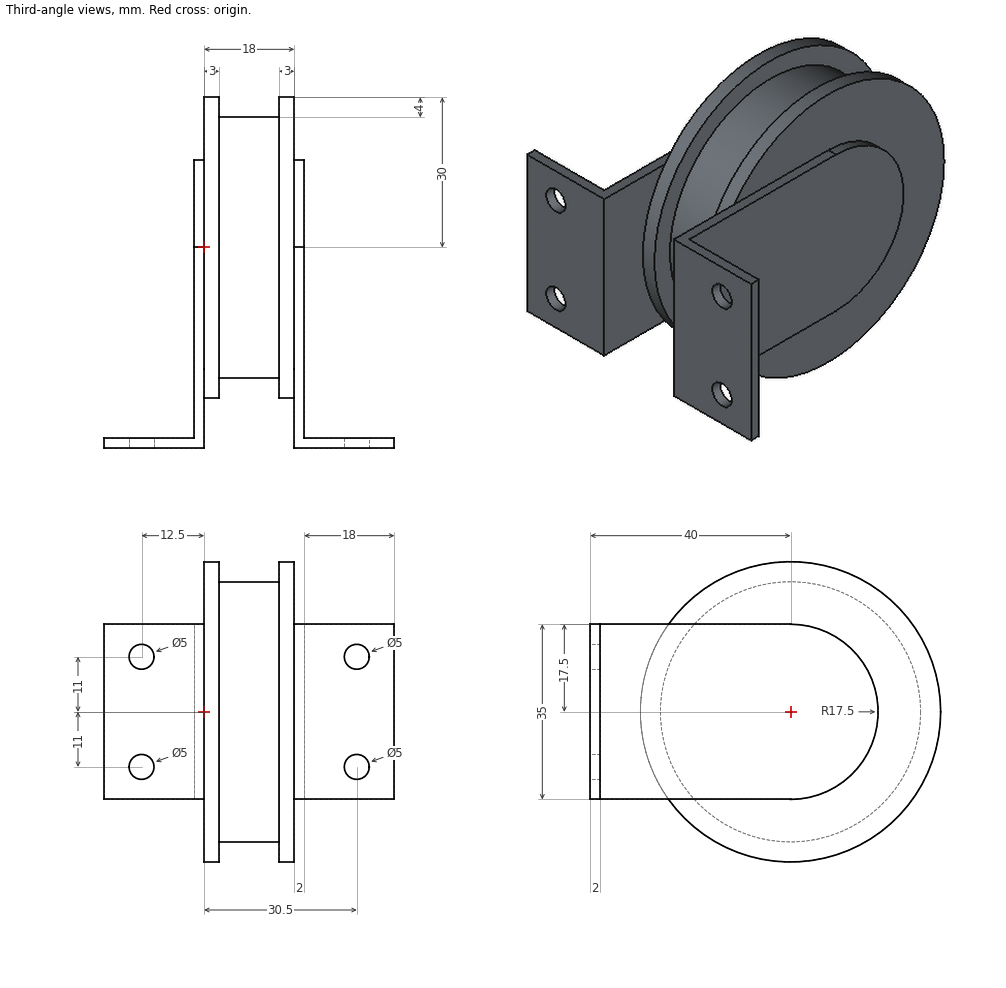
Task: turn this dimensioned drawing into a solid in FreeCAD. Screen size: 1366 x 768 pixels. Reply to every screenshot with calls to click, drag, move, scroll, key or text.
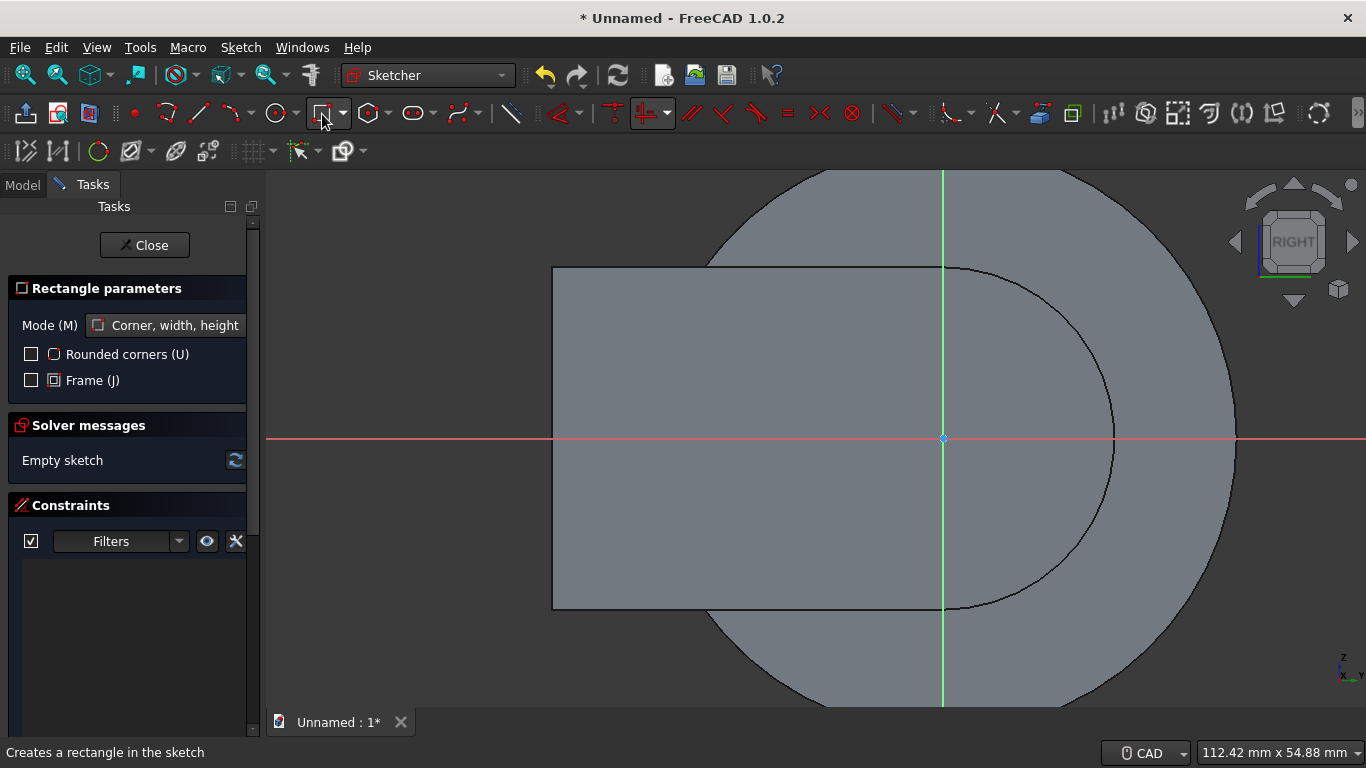
click(552, 267)
click(571, 610)
key(Escape)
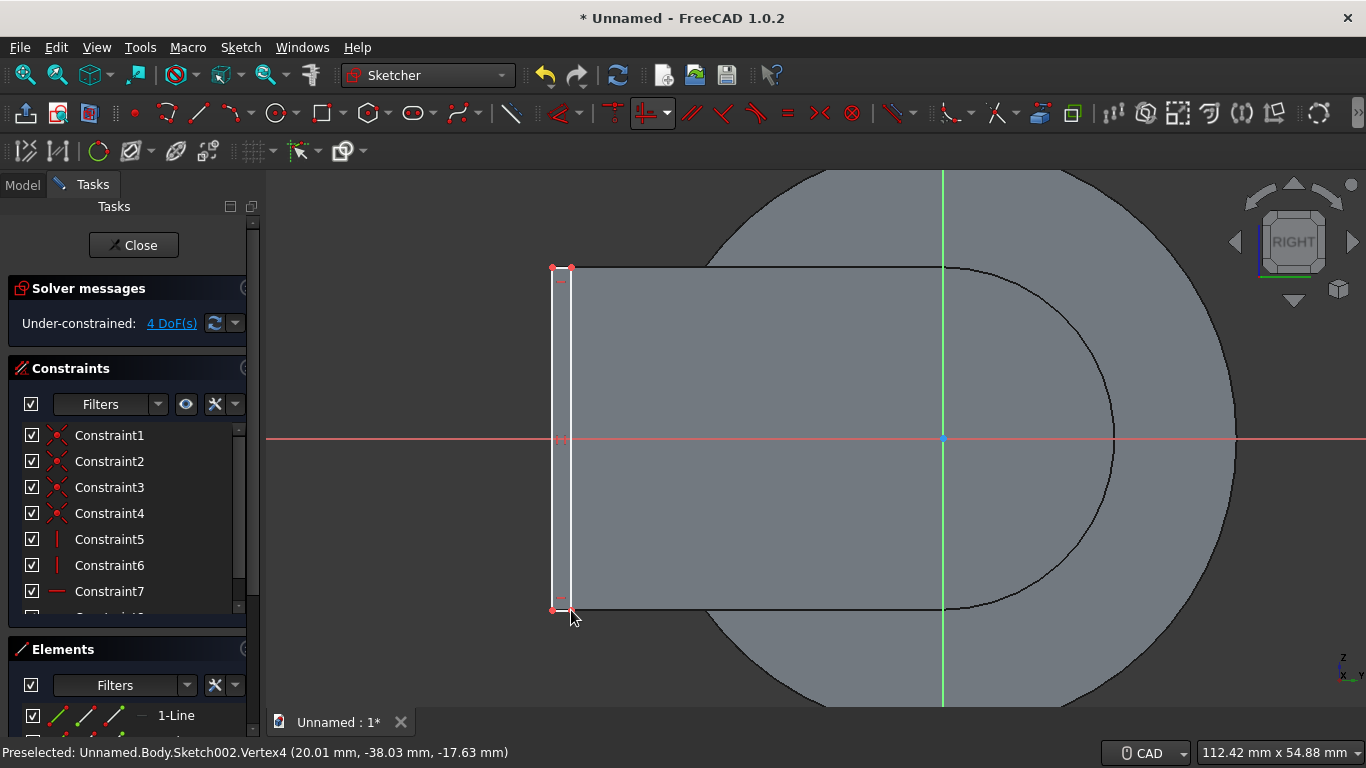
click(558, 114)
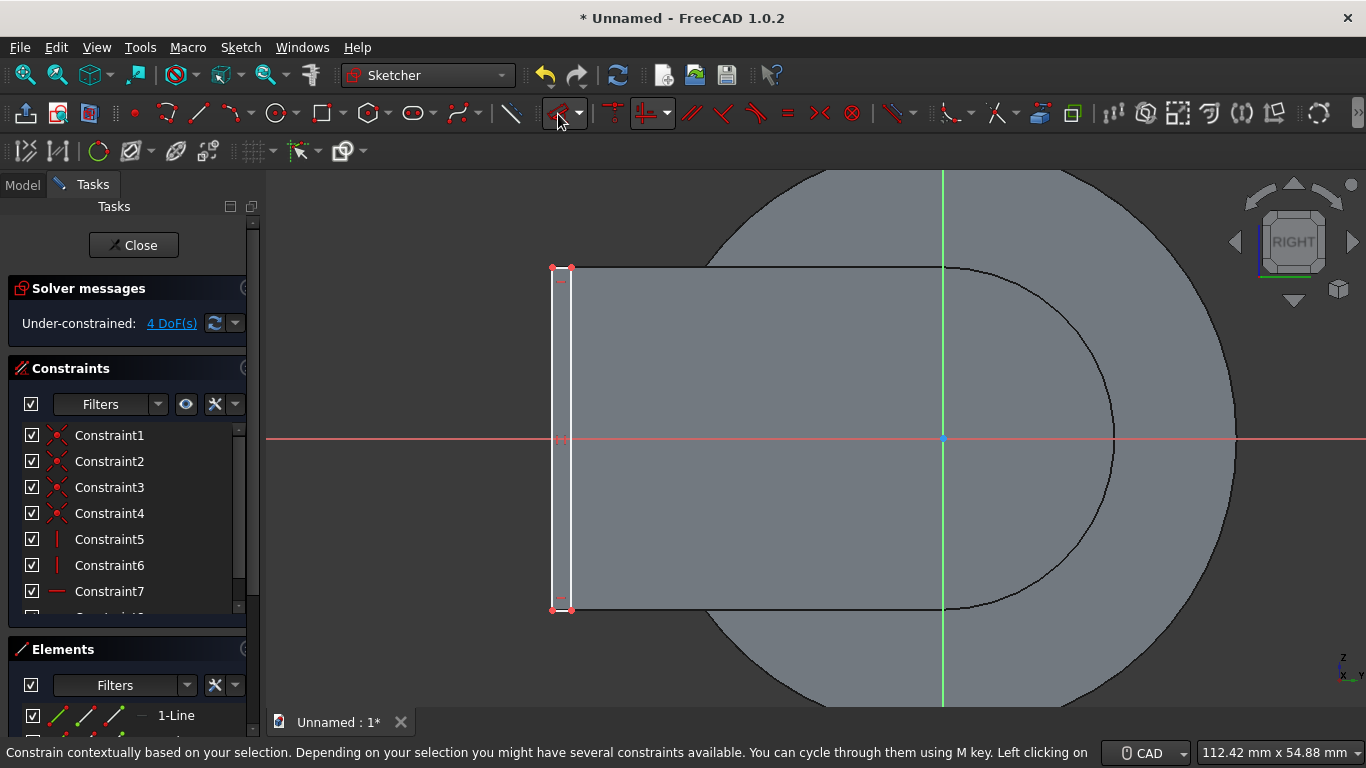
scroll(561, 611, up, 4)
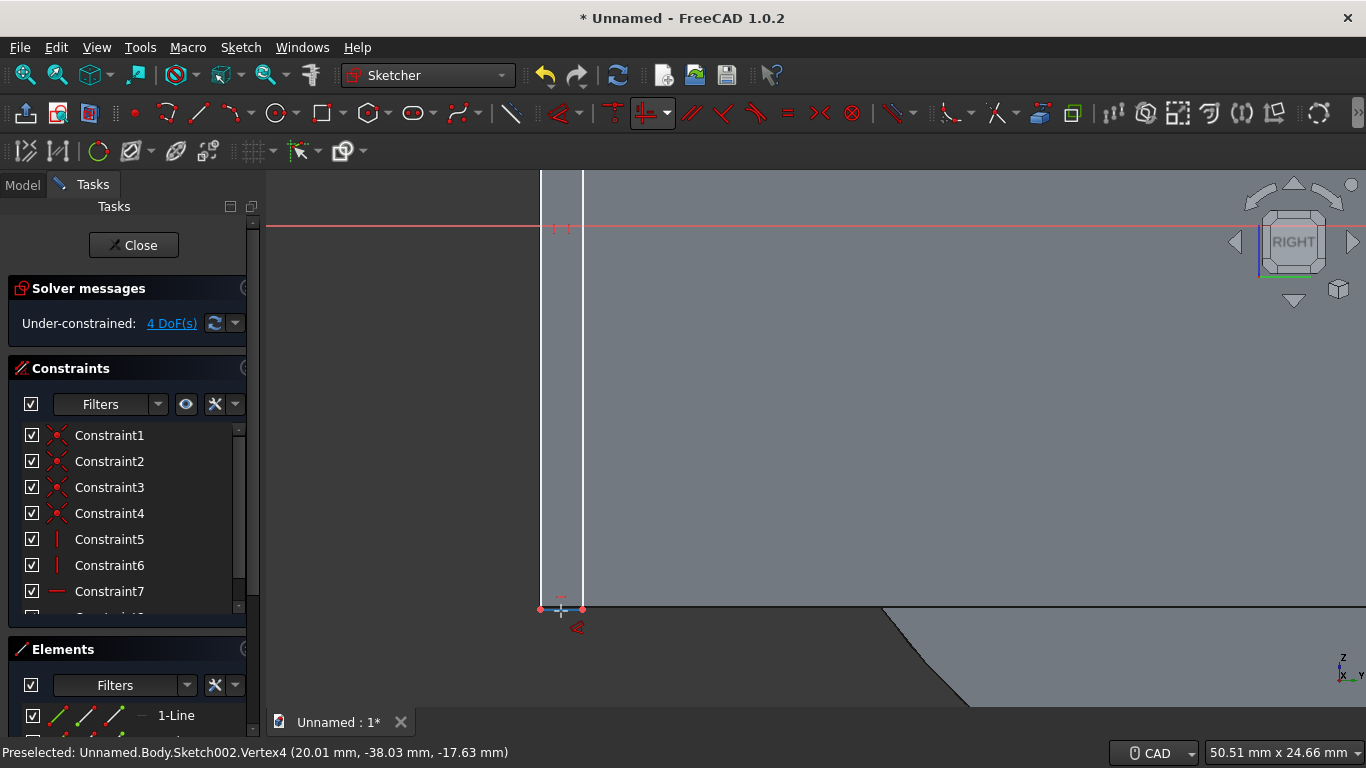
click(562, 610)
click(562, 644)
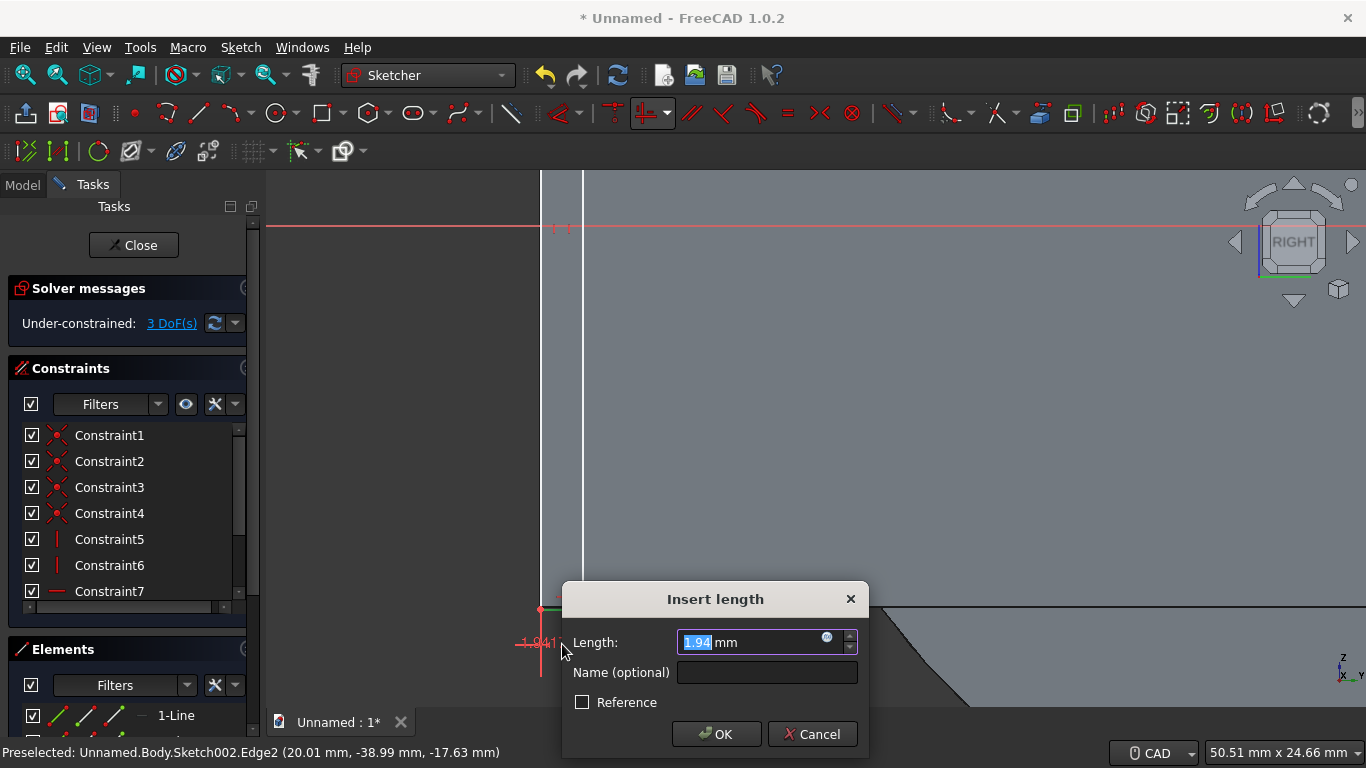
text(2)
key(Return)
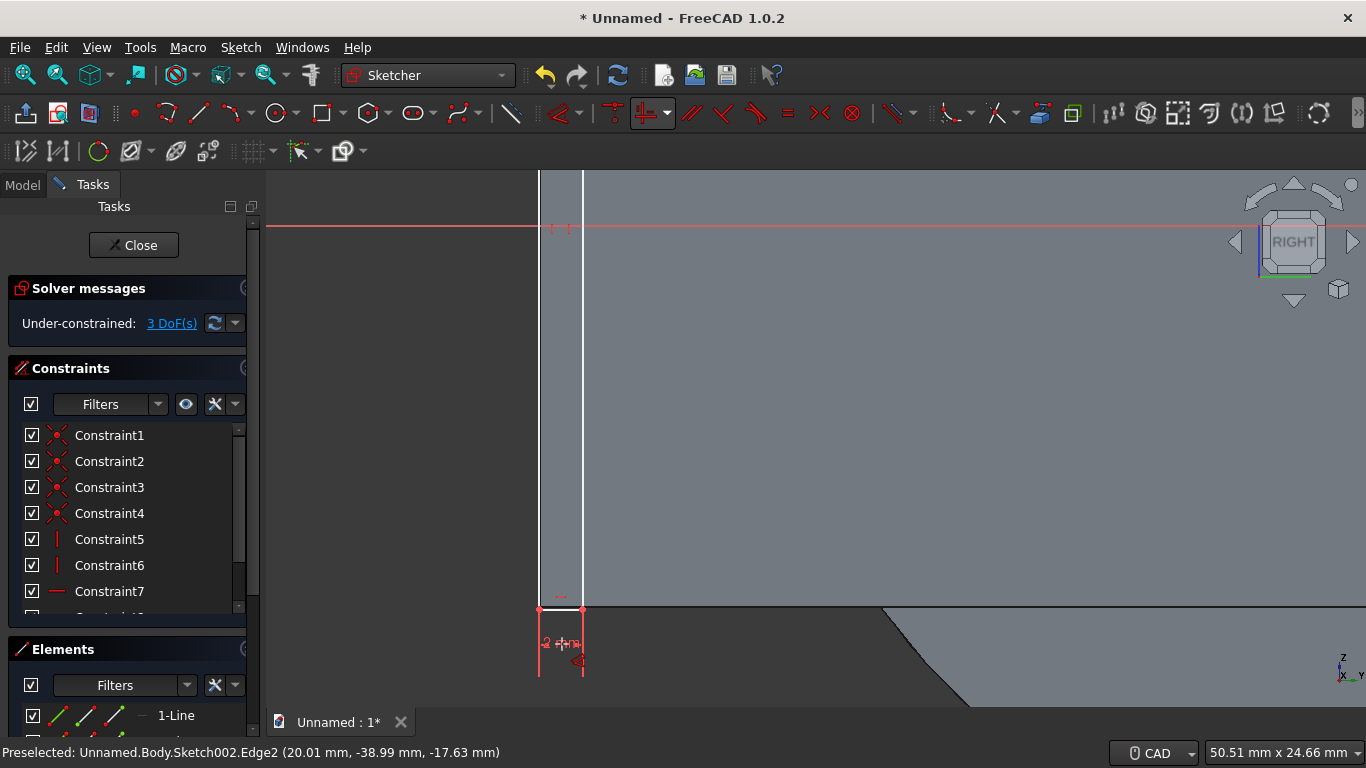
click(539, 381)
click(505, 404)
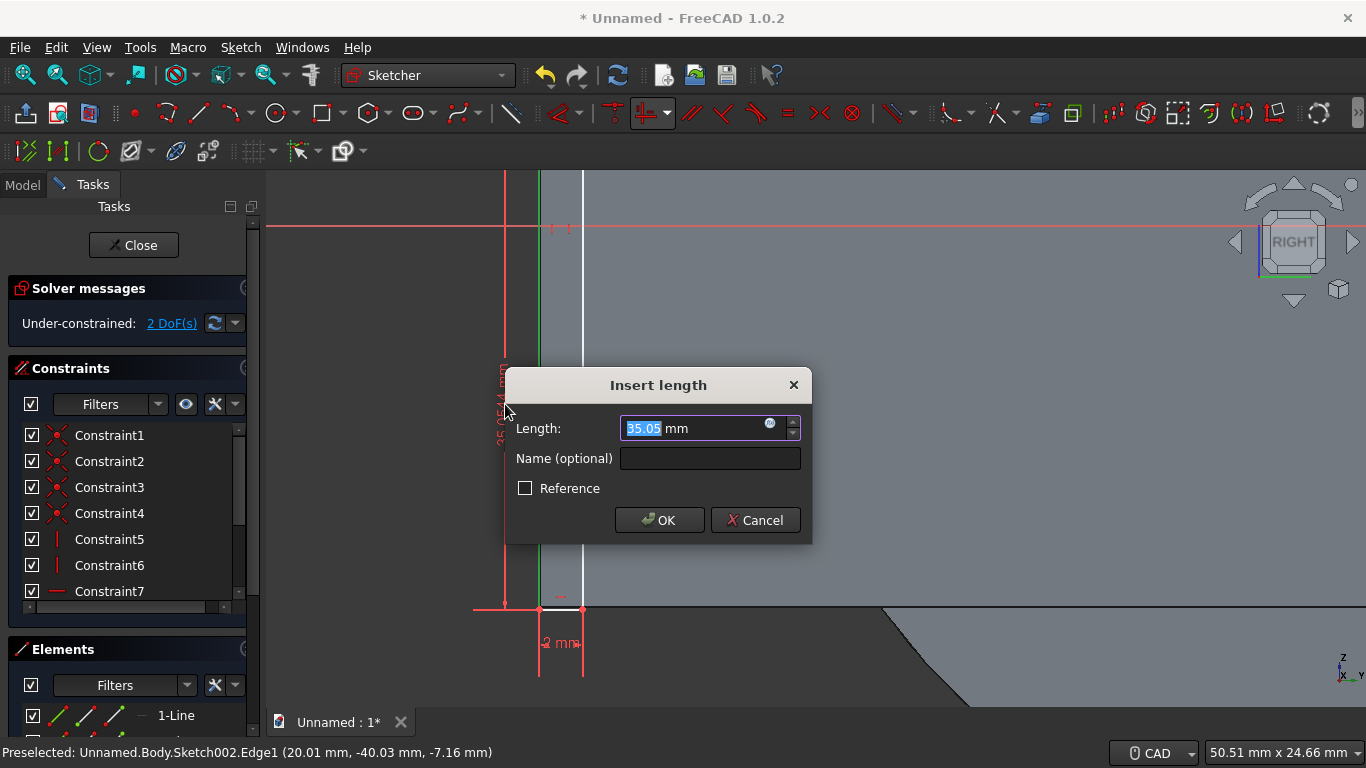
text(35)
key(Return)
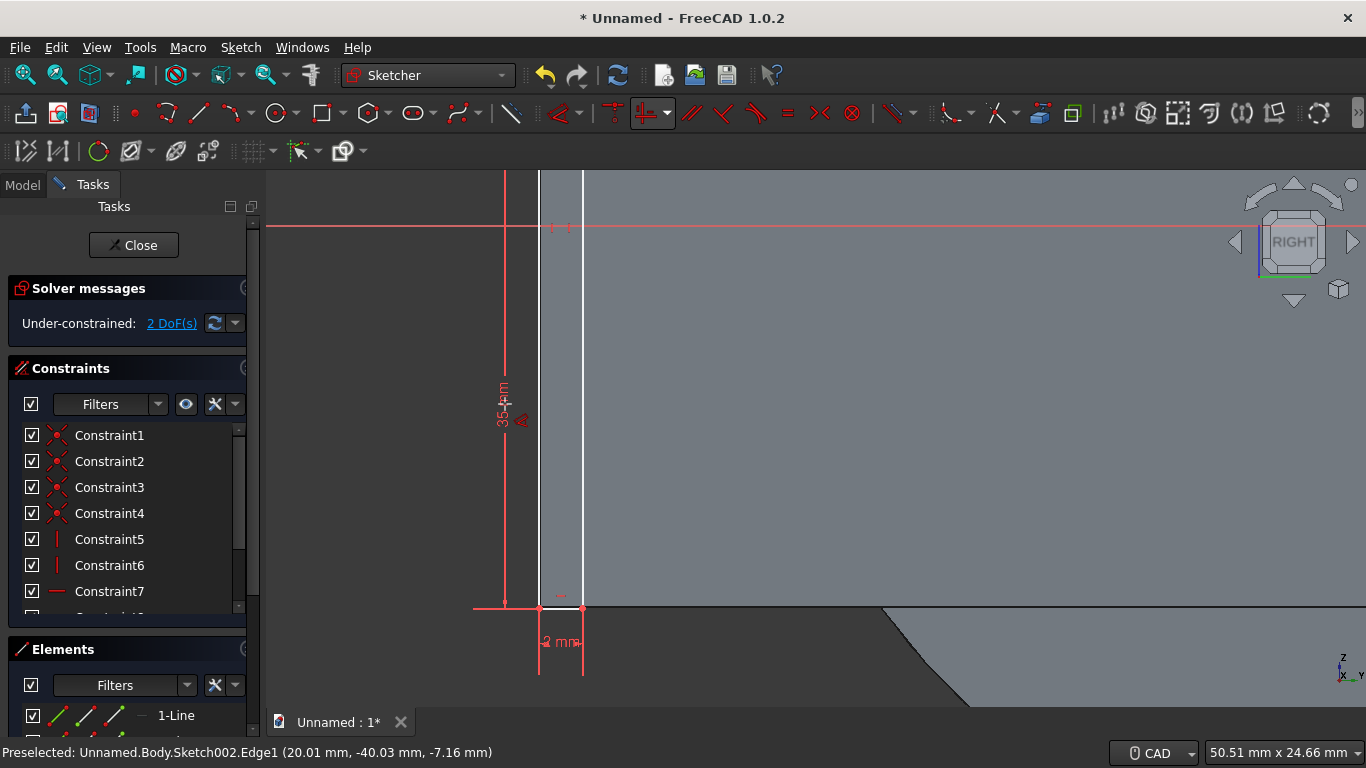
scroll(561, 612, down, 4)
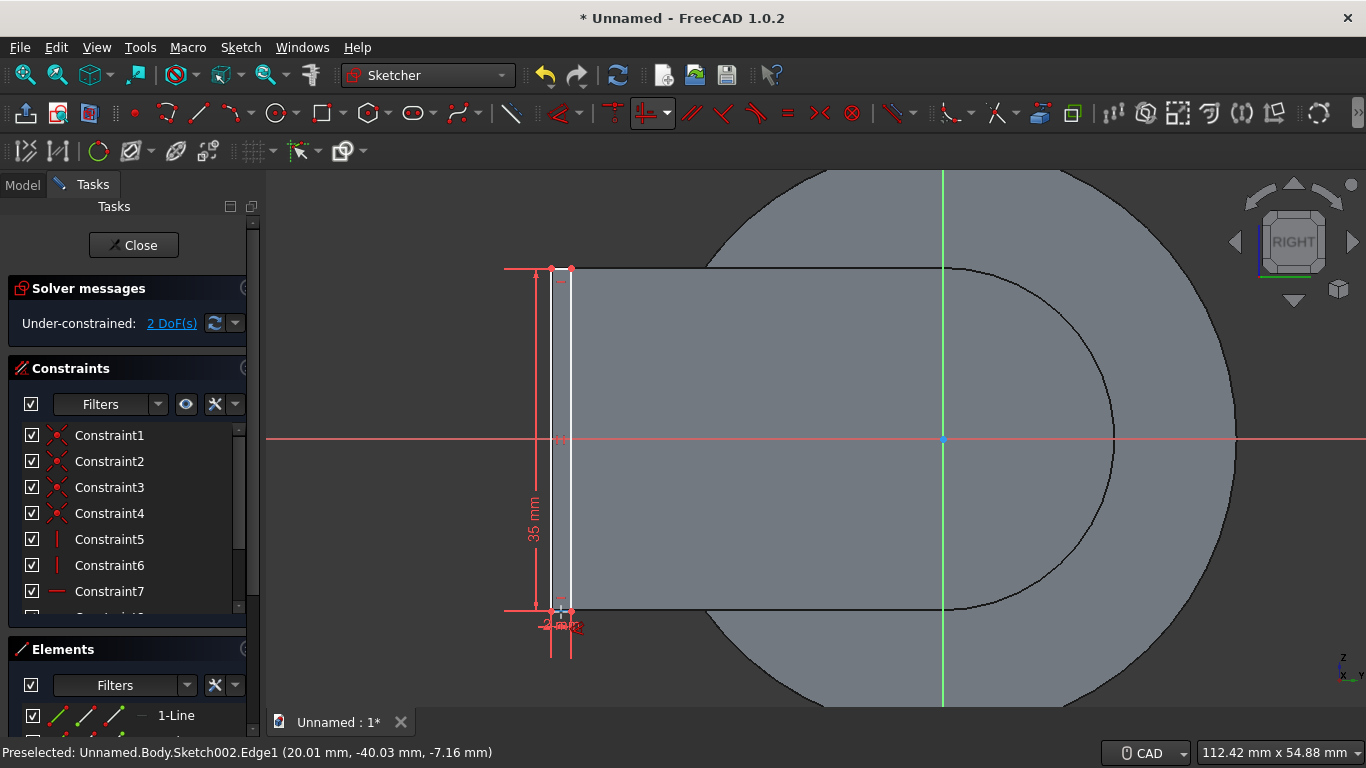
click(551, 269)
click(747, 235)